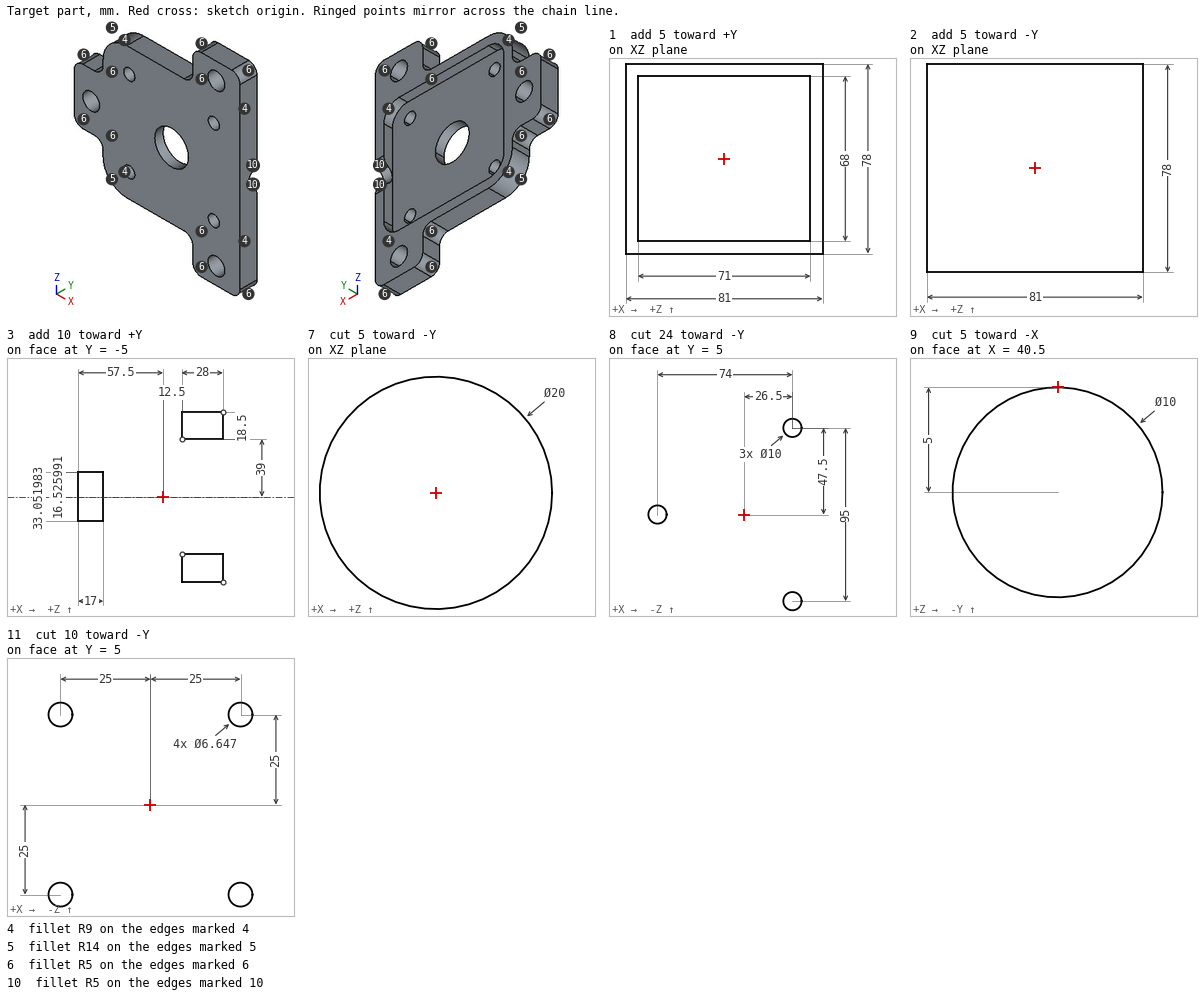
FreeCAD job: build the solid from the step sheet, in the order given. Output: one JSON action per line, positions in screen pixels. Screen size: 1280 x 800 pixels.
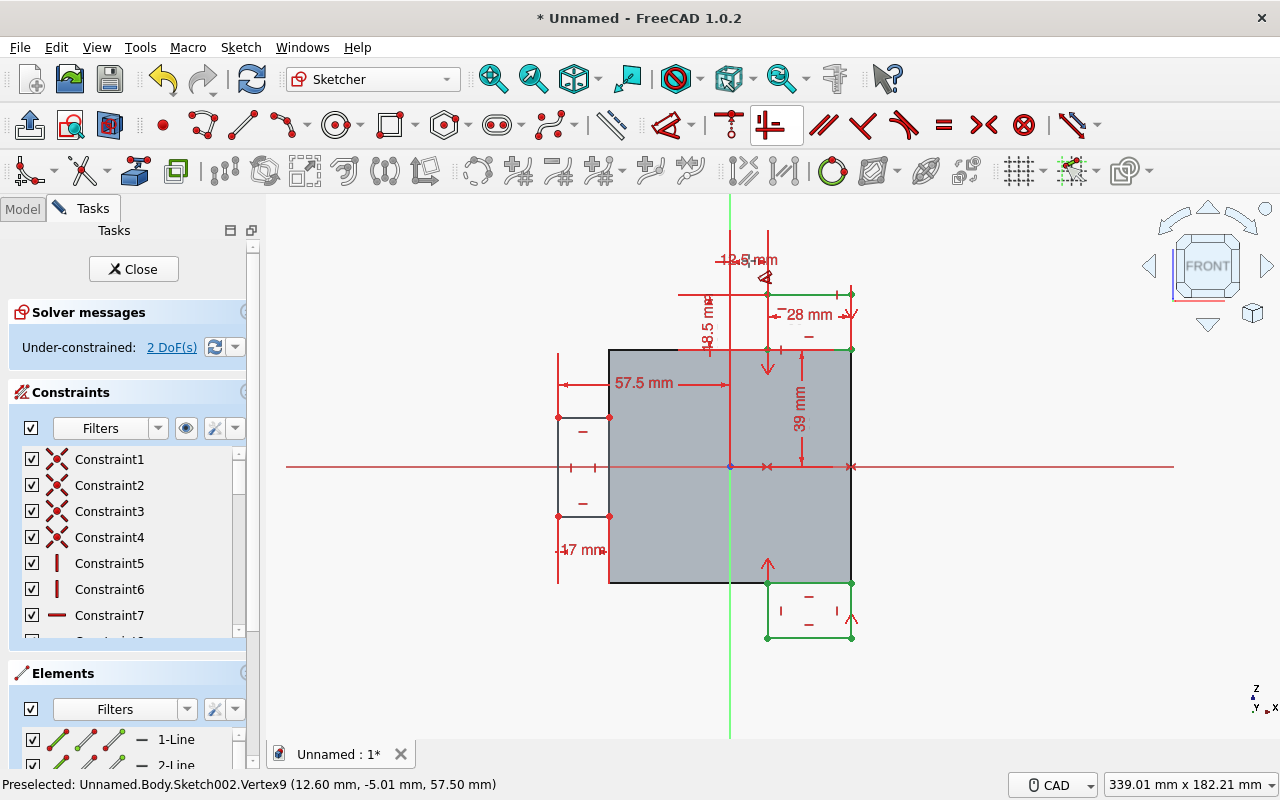
{"action": "left_click", "coordinate": [558, 448]}
{"action": "left_click", "coordinate": [524, 445]}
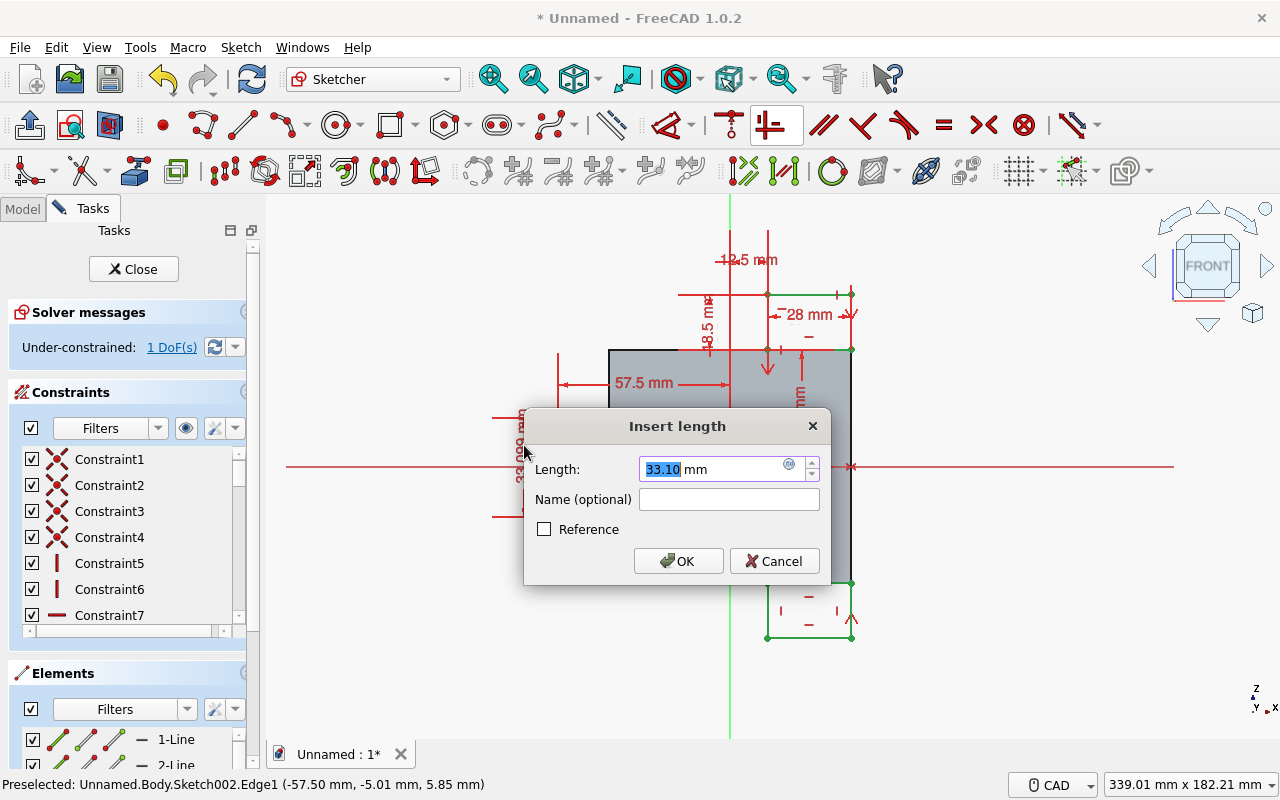
{"action": "type", "text": "33.051983"}
{"action": "key", "text": "Return"}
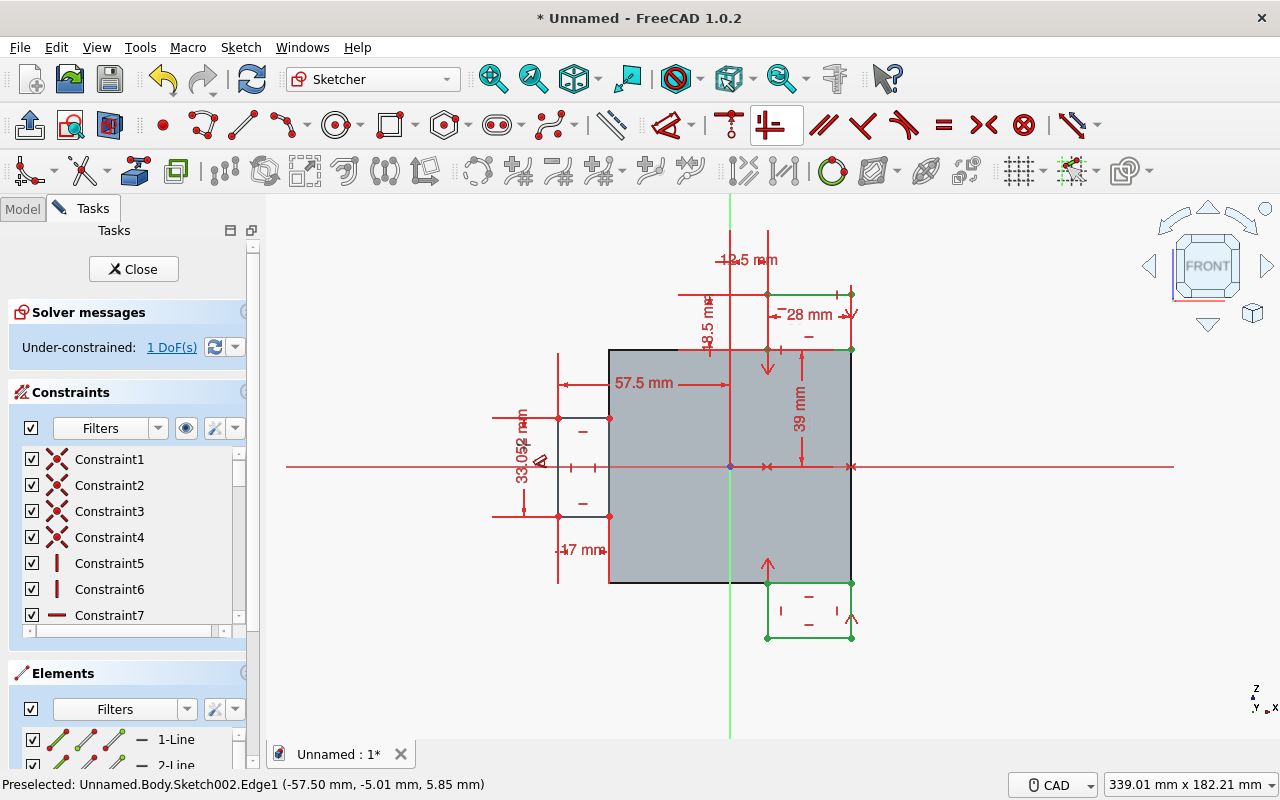
{"action": "left_click", "coordinate": [558, 418]}
{"action": "left_click", "coordinate": [764, 442]}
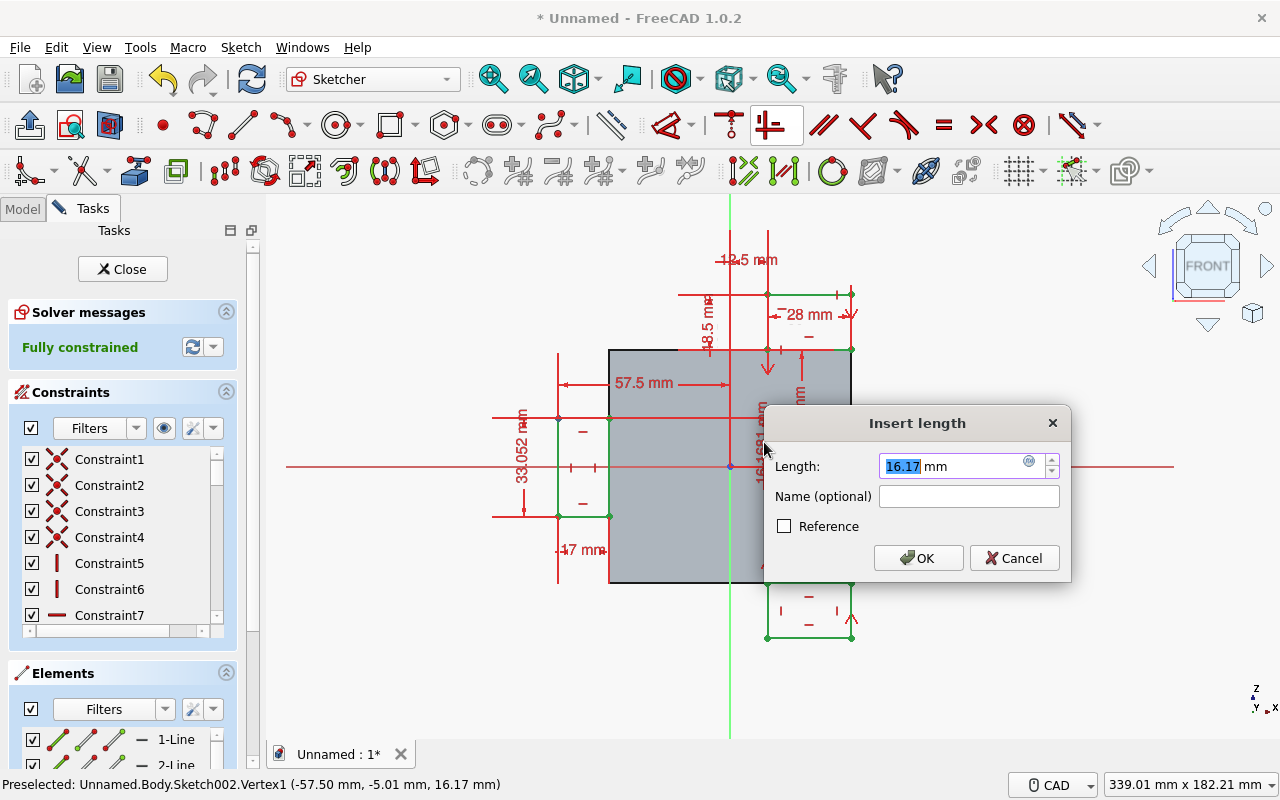
{"action": "type", "text": "16.525991"}
{"action": "key", "text": "Return"}
{"action": "key", "text": "Escape"}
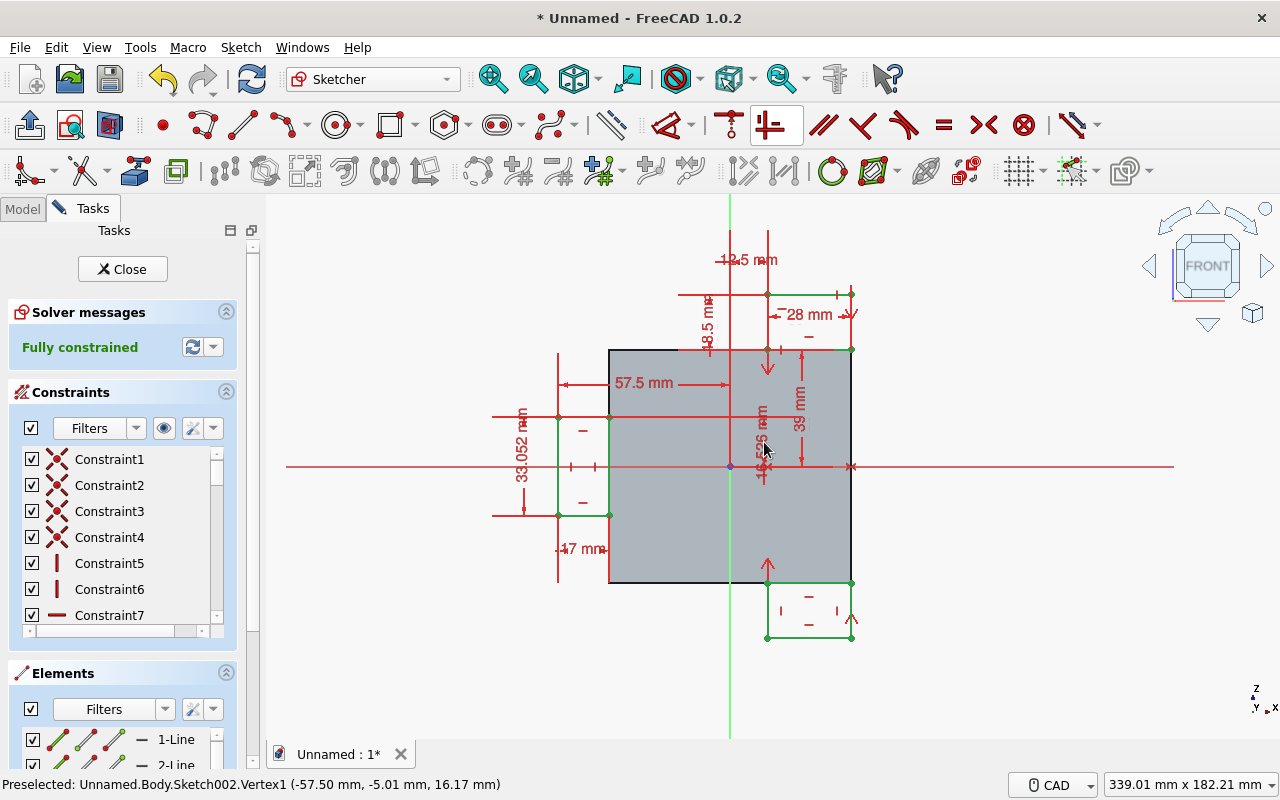
{"action": "left_click", "coordinate": [123, 269]}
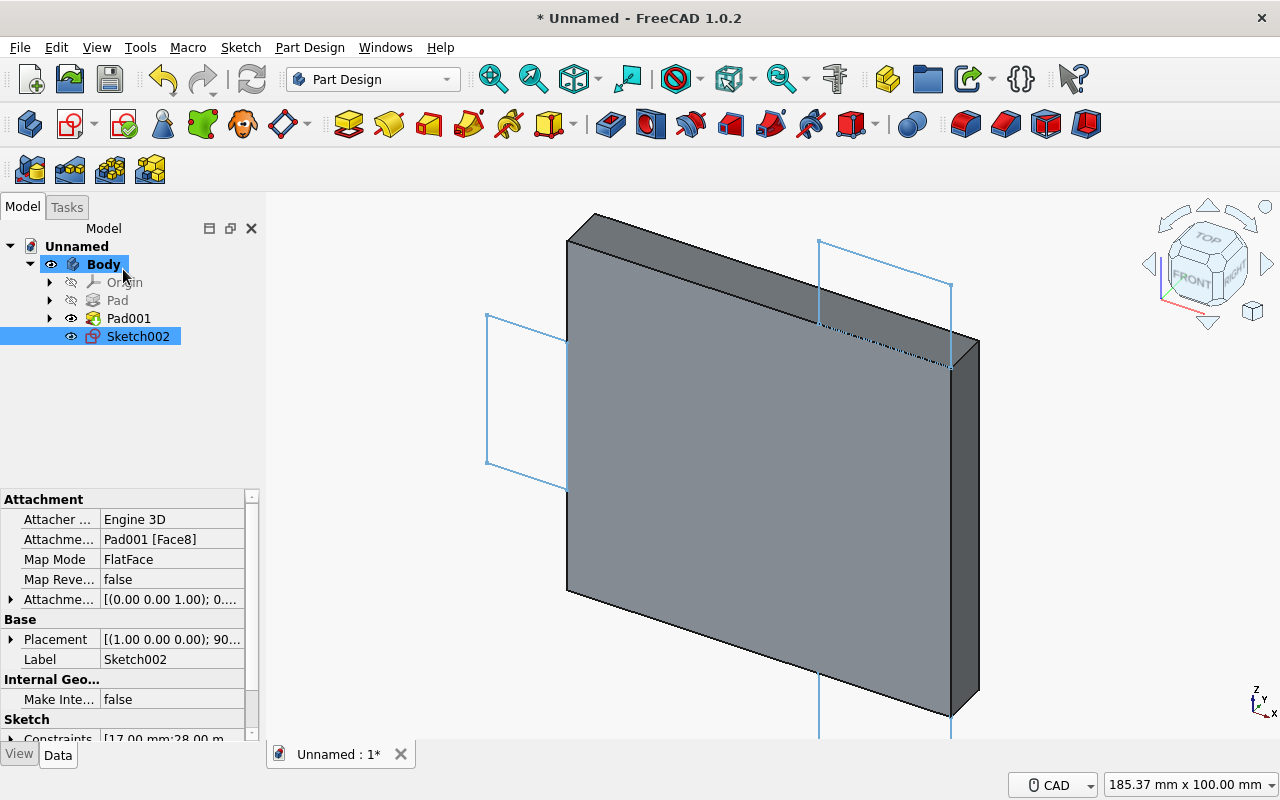
{"action": "left_click", "coordinate": [350, 124]}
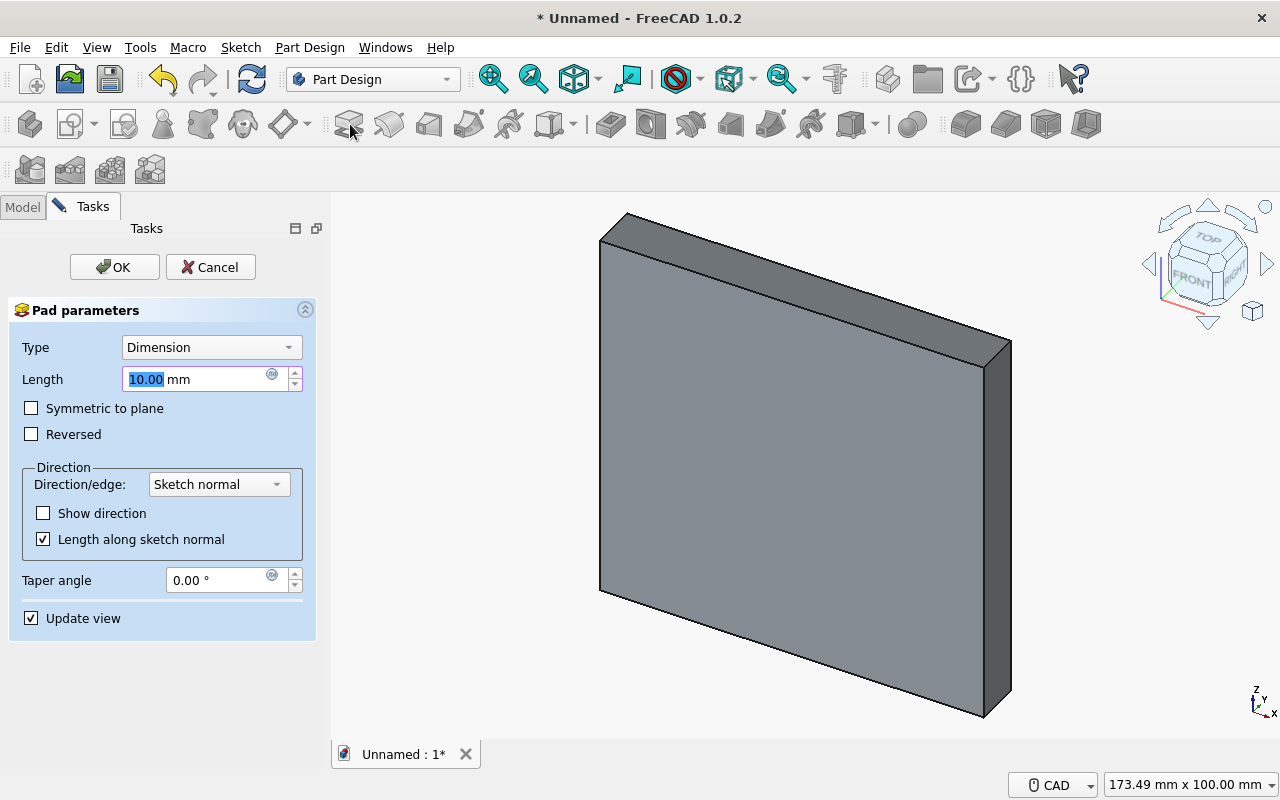
{"action": "type", "text": "10"}
{"action": "key", "text": "Tab"}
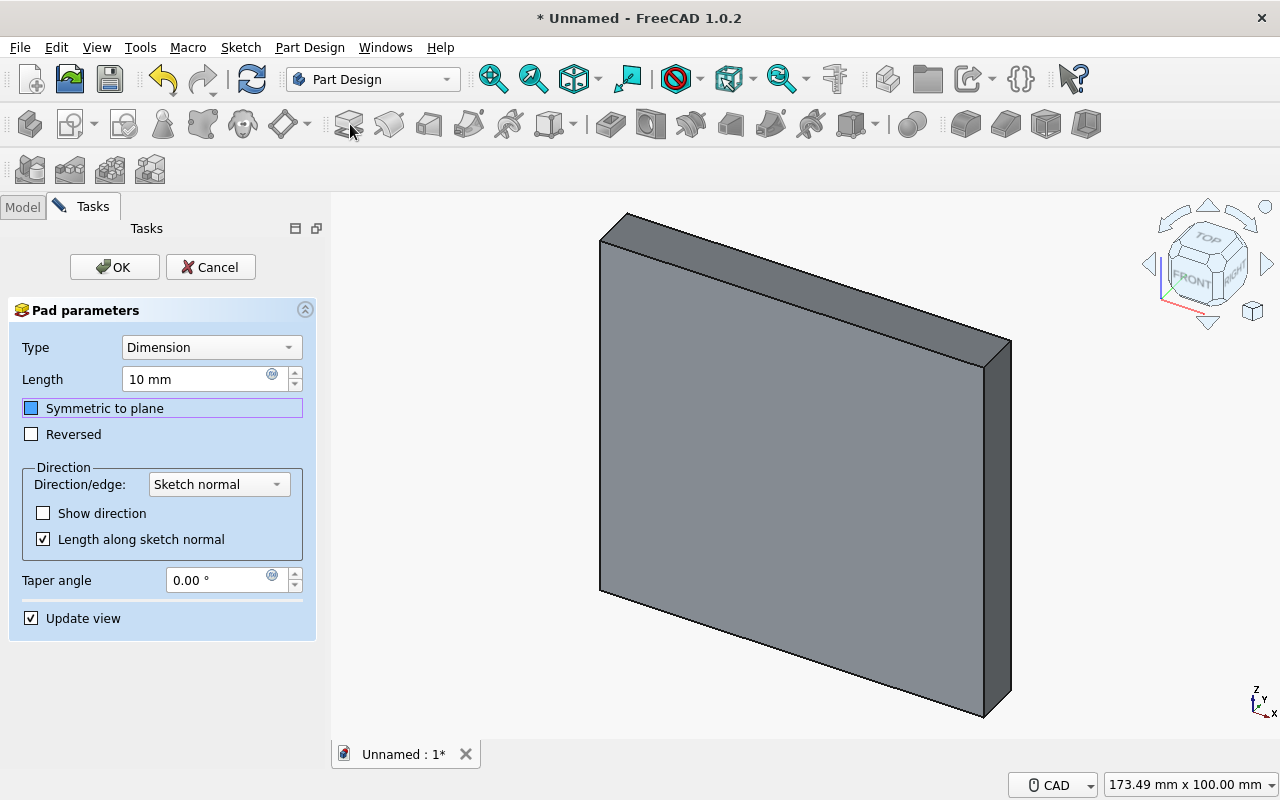
{"action": "left_click", "coordinate": [30, 434]}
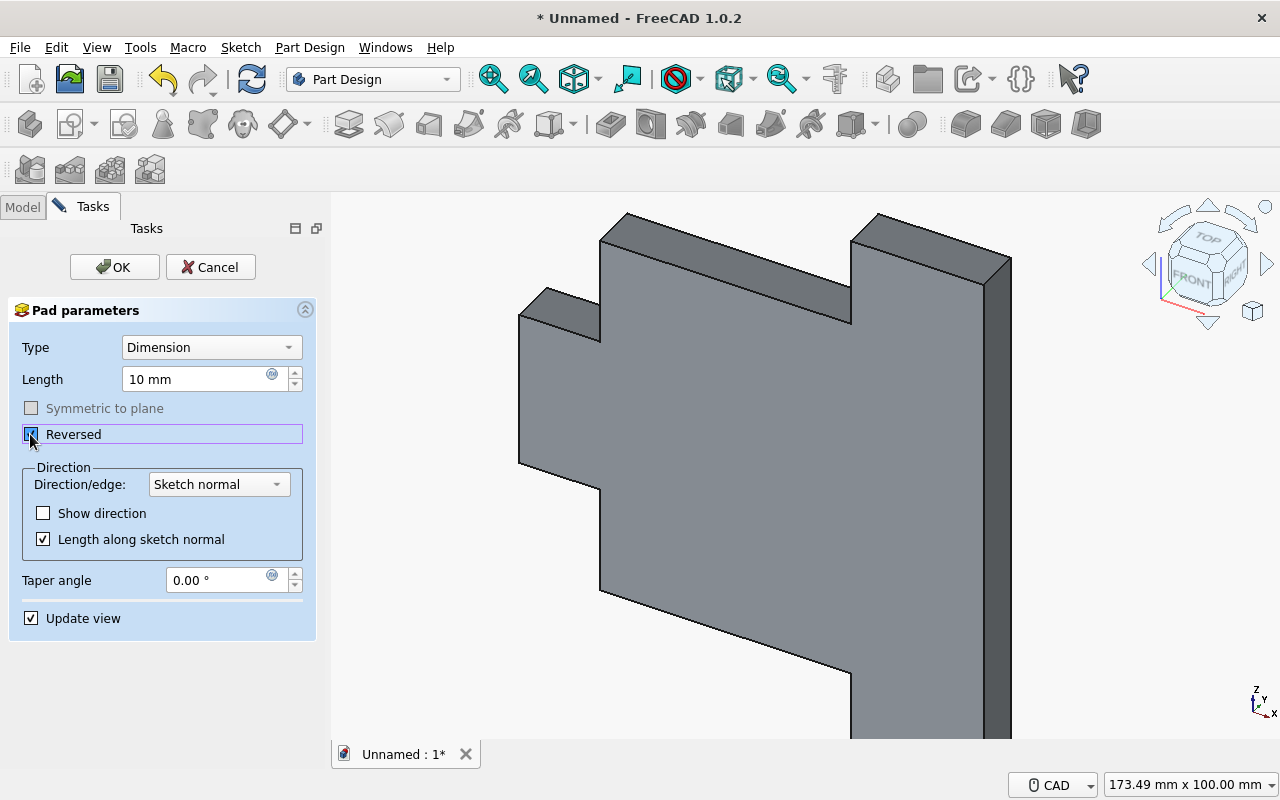
{"action": "left_click", "coordinate": [115, 267]}